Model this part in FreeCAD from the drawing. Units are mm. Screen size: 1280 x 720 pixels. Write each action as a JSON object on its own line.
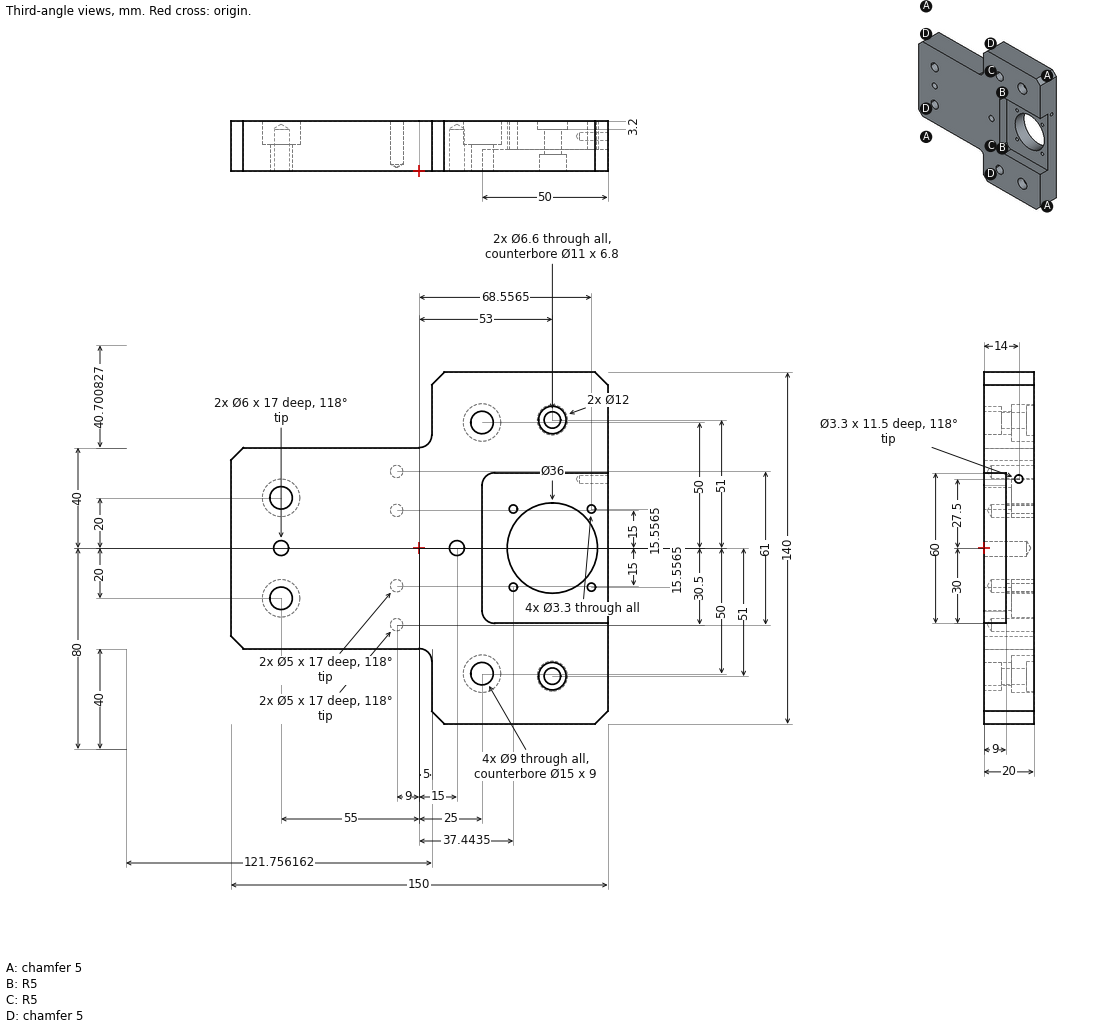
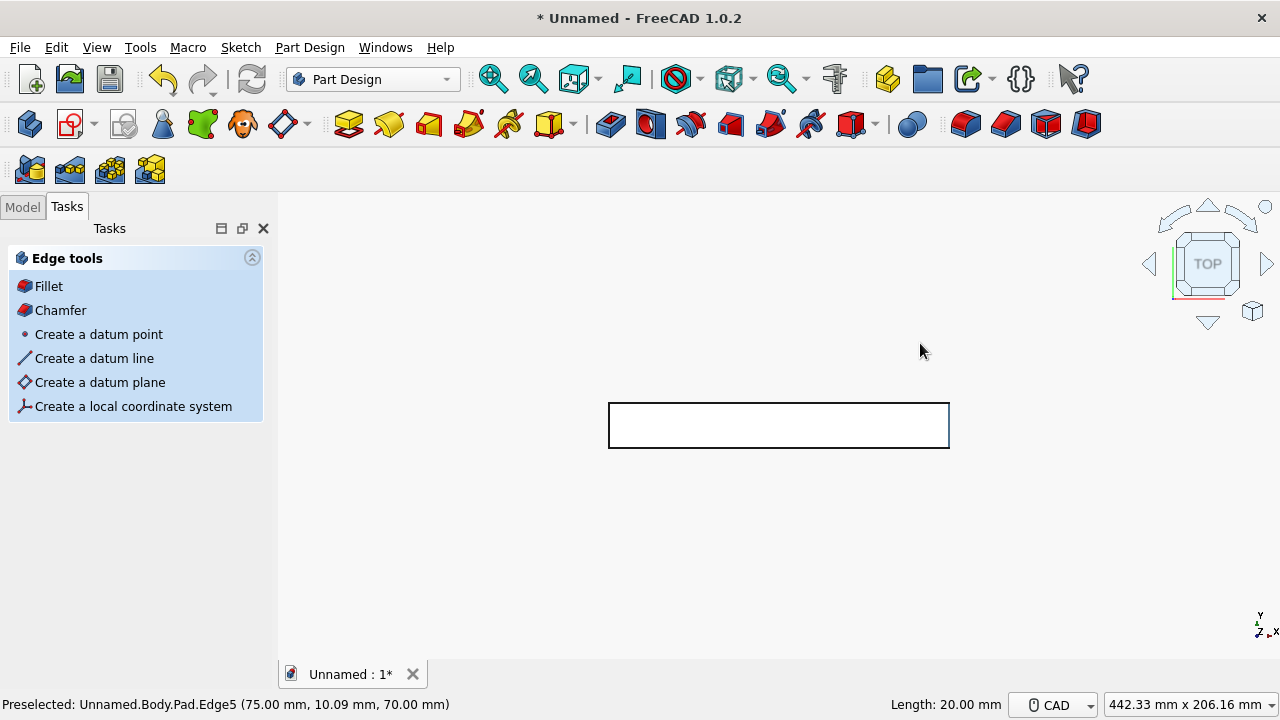
{"action": "left_click", "coordinate": [494, 80]}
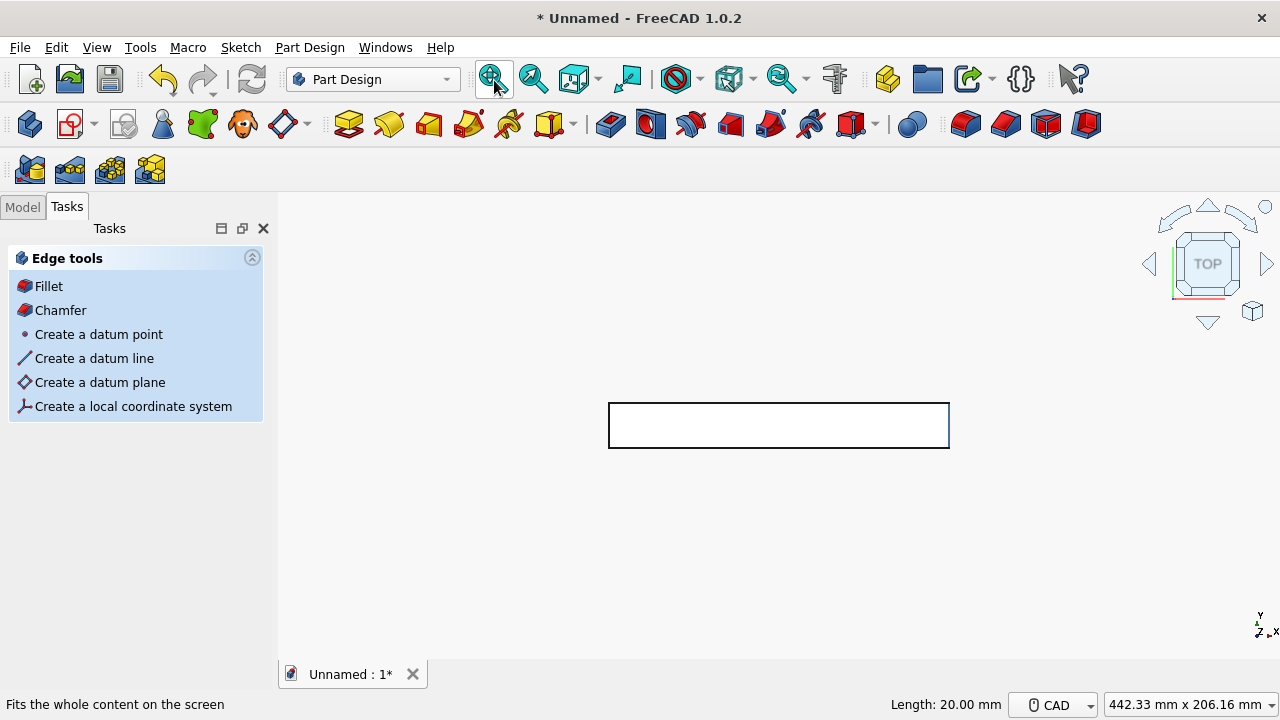
{"action": "left_click", "coordinate": [609, 424], "text": "ctrl"}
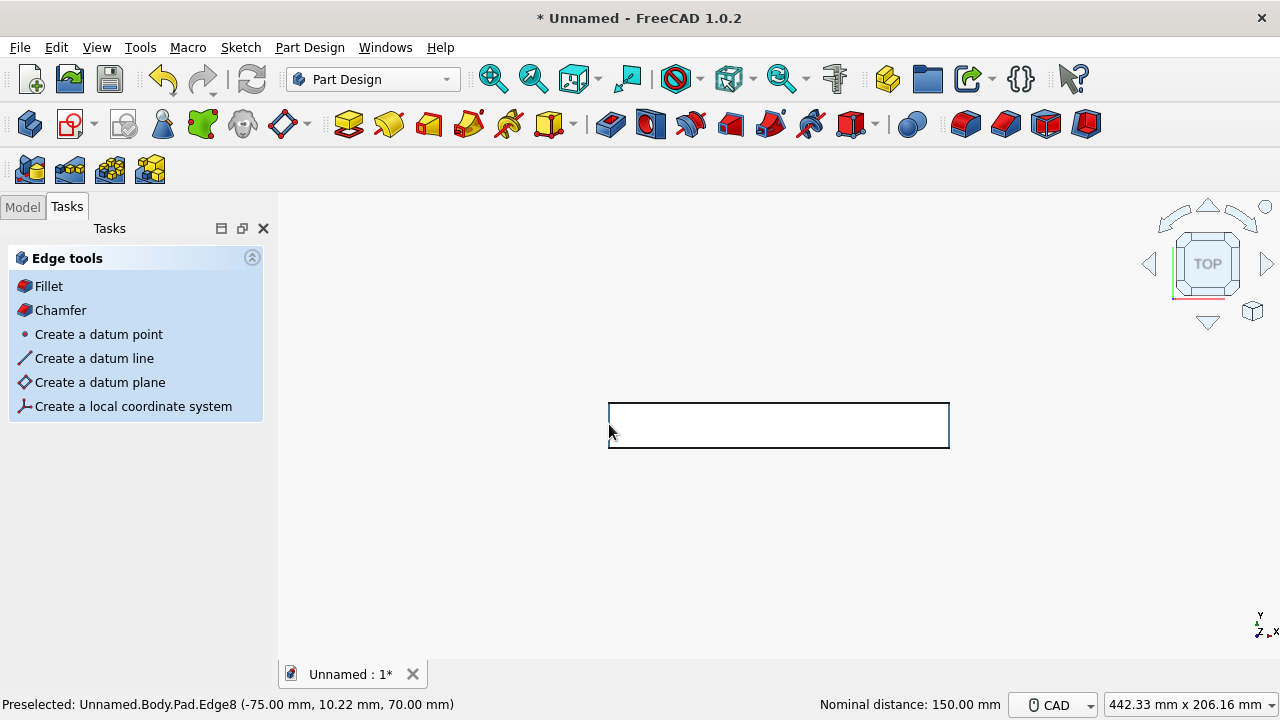
{"action": "key", "text": "1"}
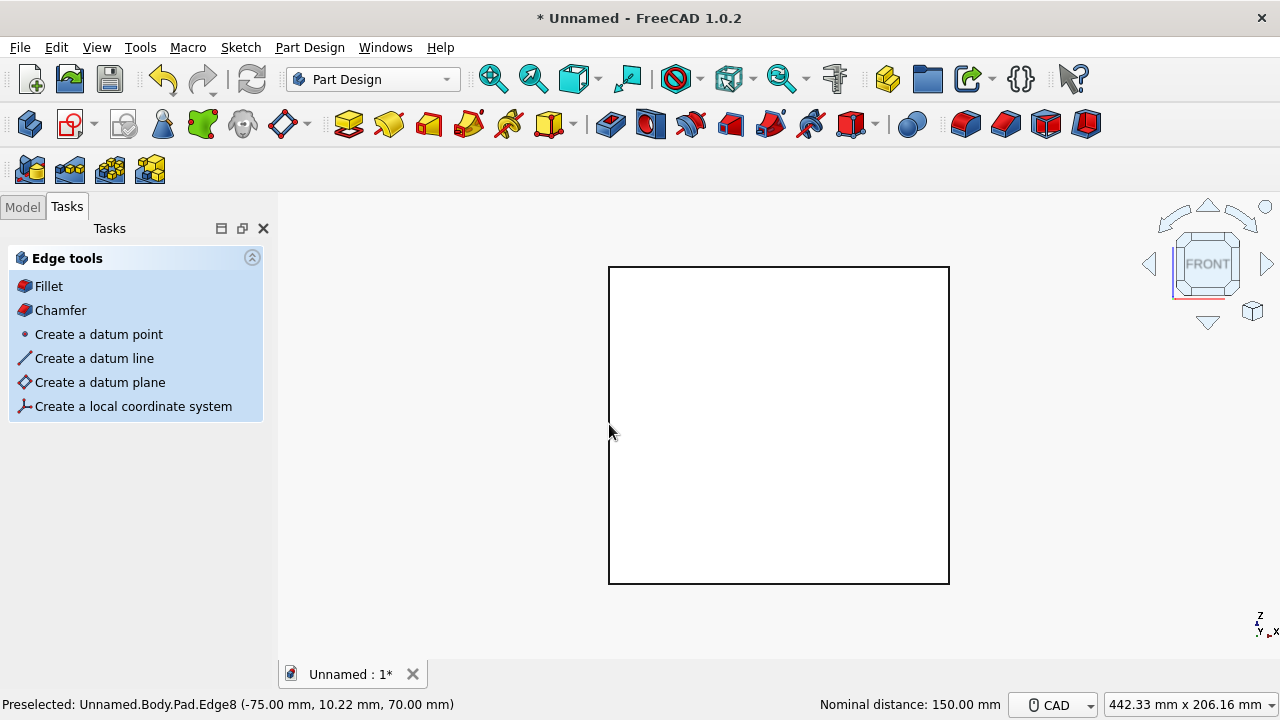
{"action": "key", "text": "3"}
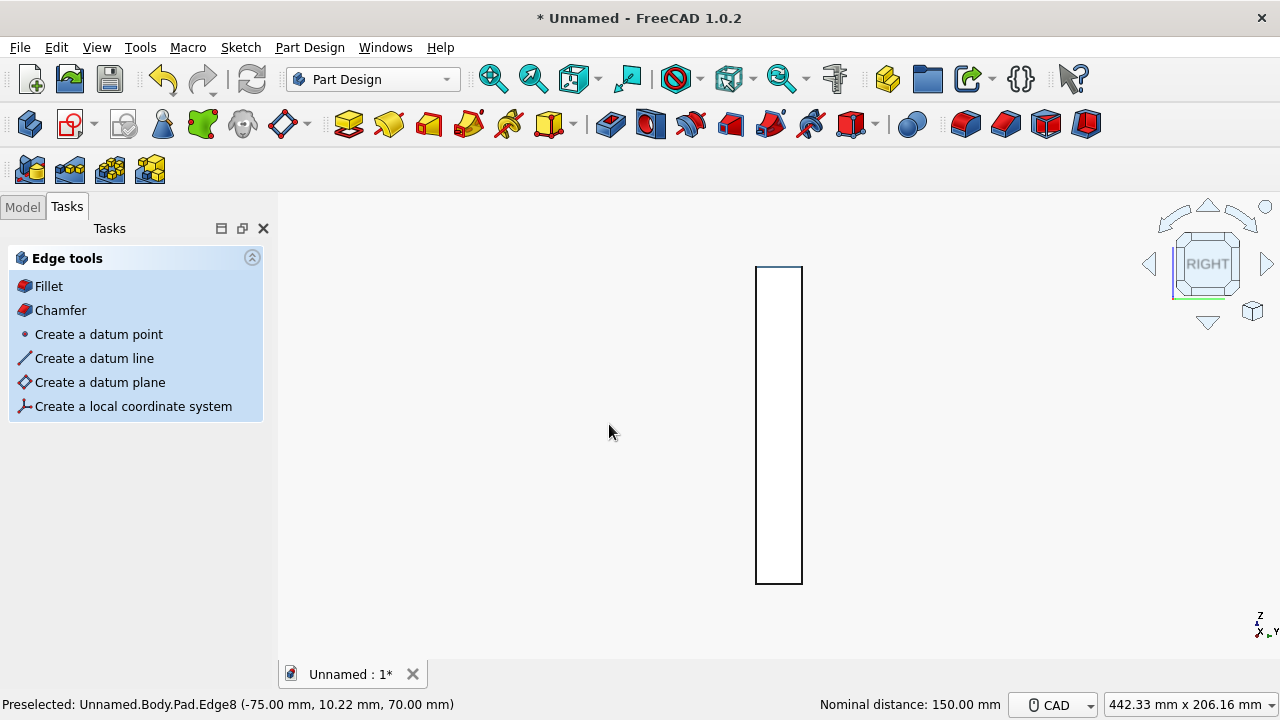
{"action": "left_click", "coordinate": [779, 583], "text": "ctrl"}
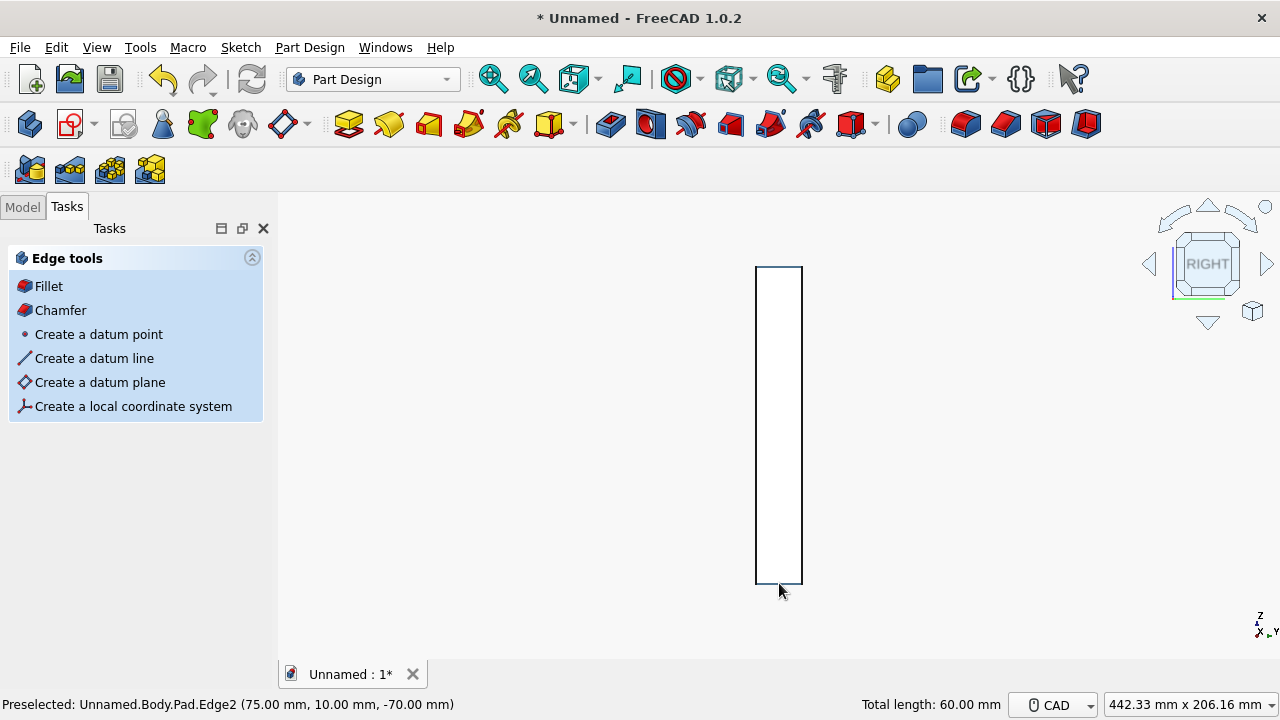
{"action": "key", "text": "5"}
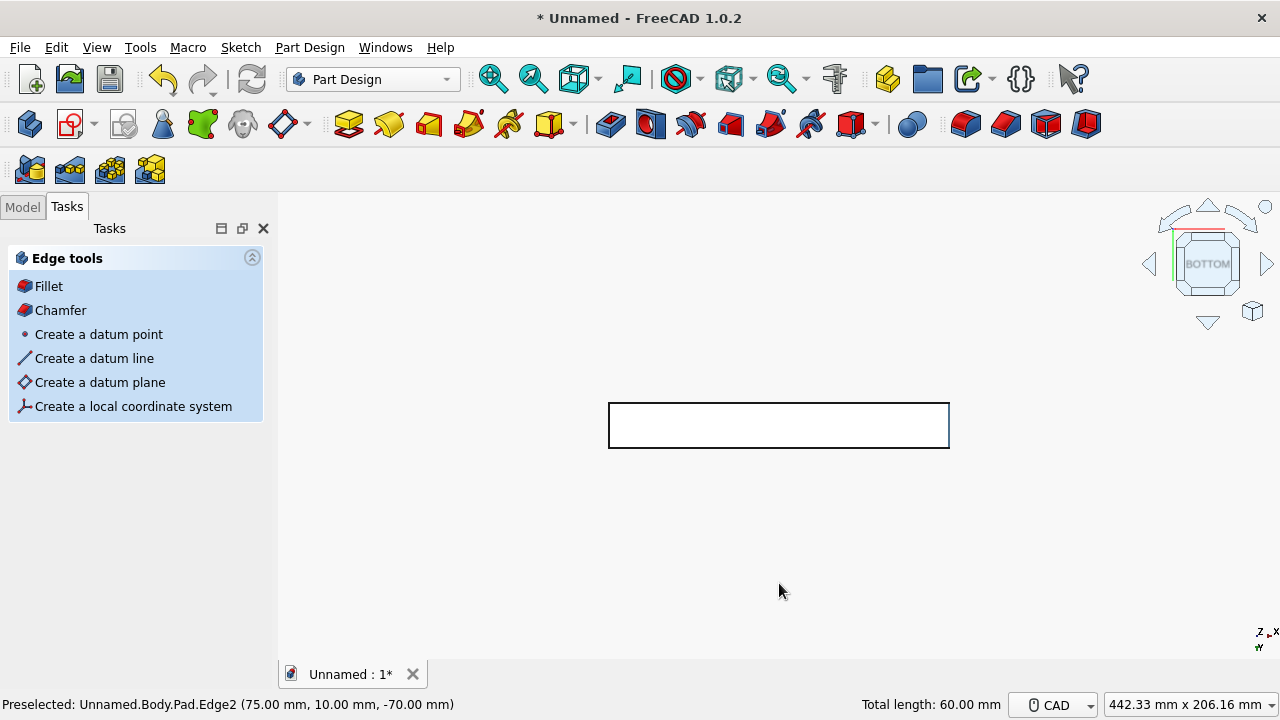
{"action": "left_click", "coordinate": [494, 80]}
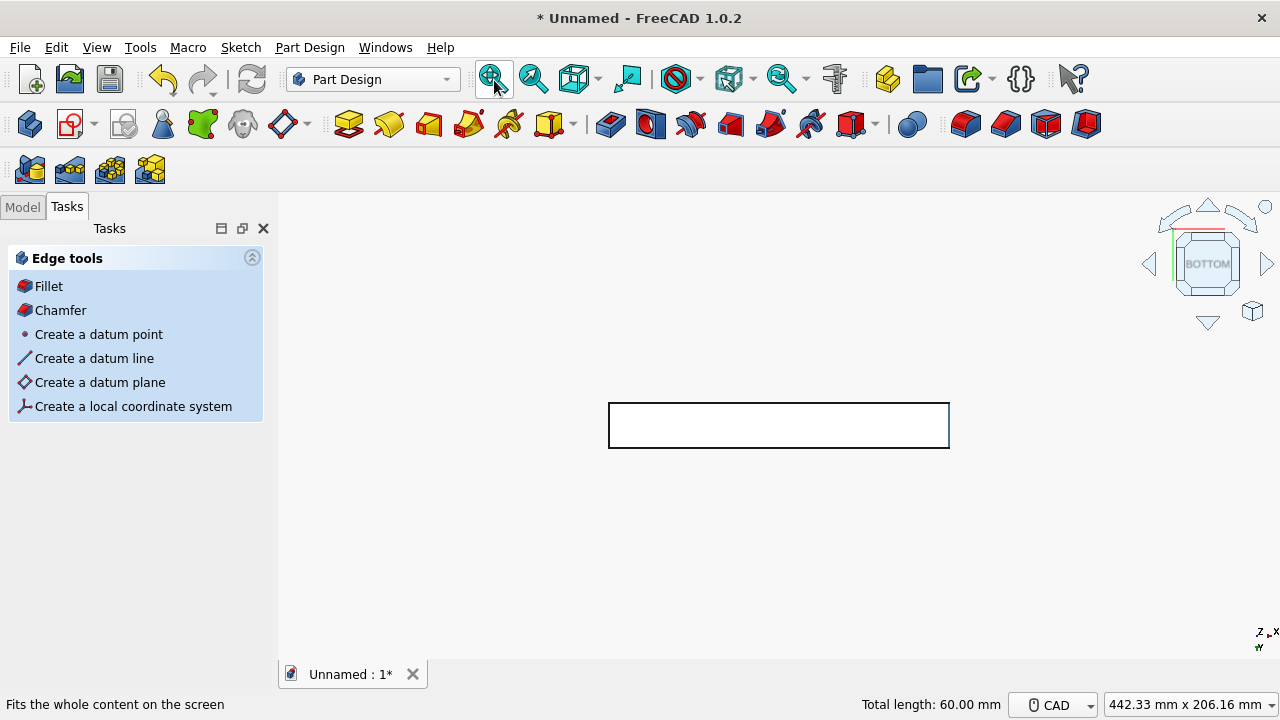
{"action": "left_click", "coordinate": [609, 424], "text": "ctrl"}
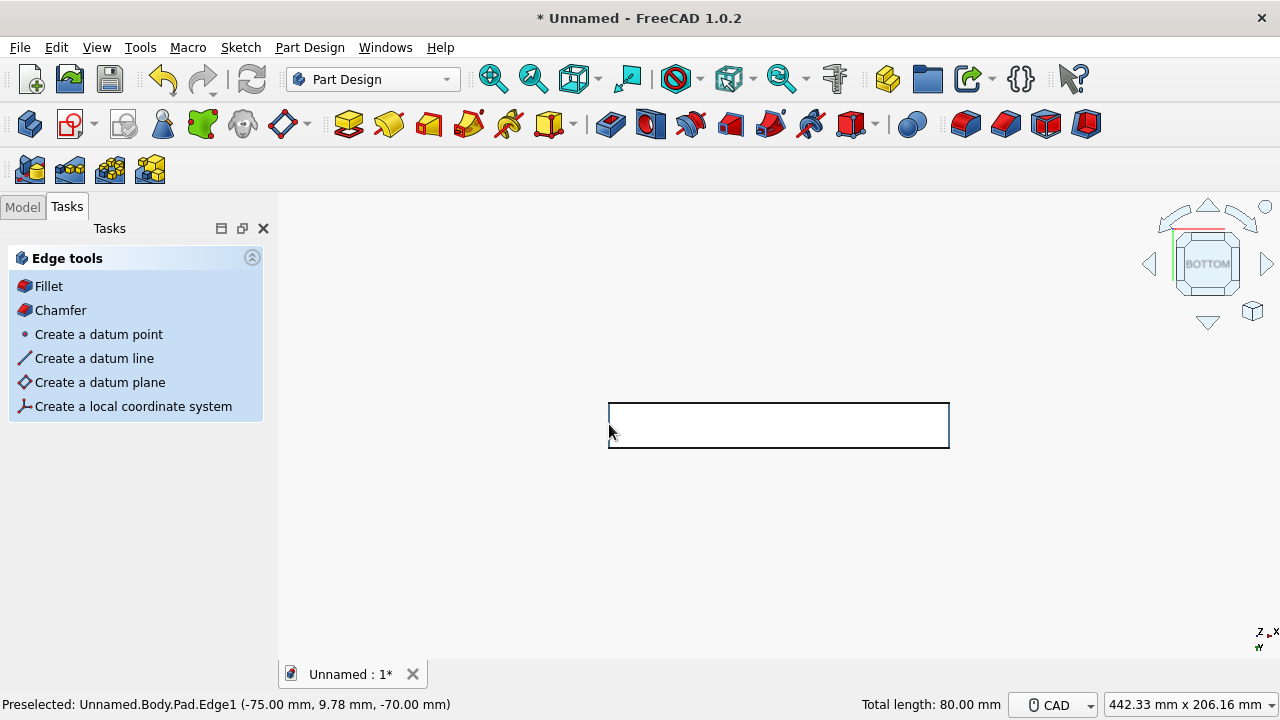
{"action": "left_click", "coordinate": [1006, 124]}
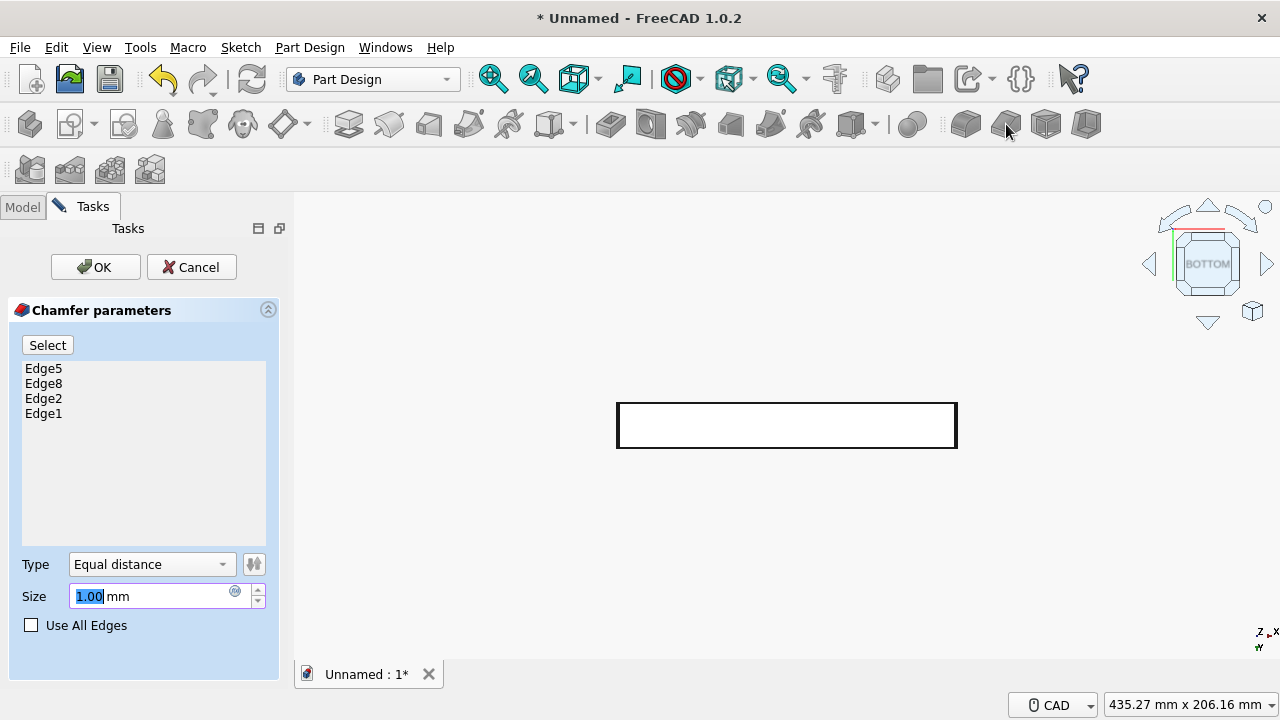
{"action": "type", "text": "5"}
{"action": "key", "text": "Tab"}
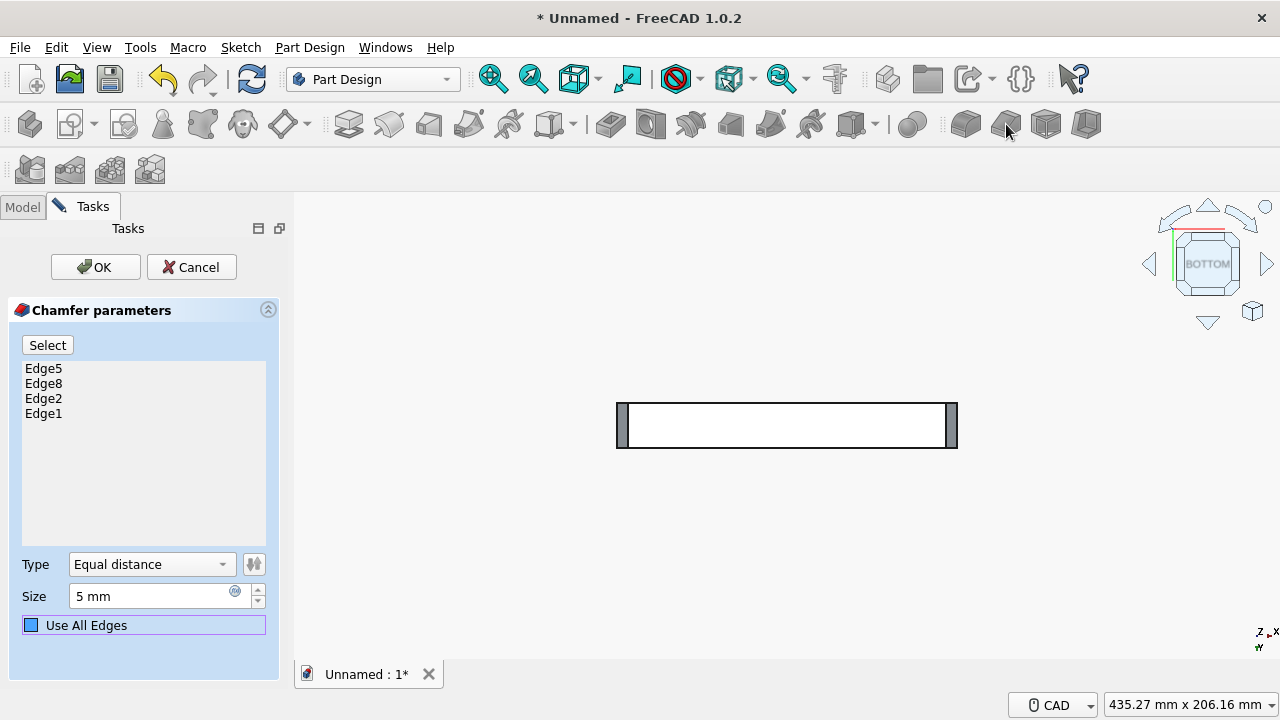
{"action": "left_click", "coordinate": [96, 267]}